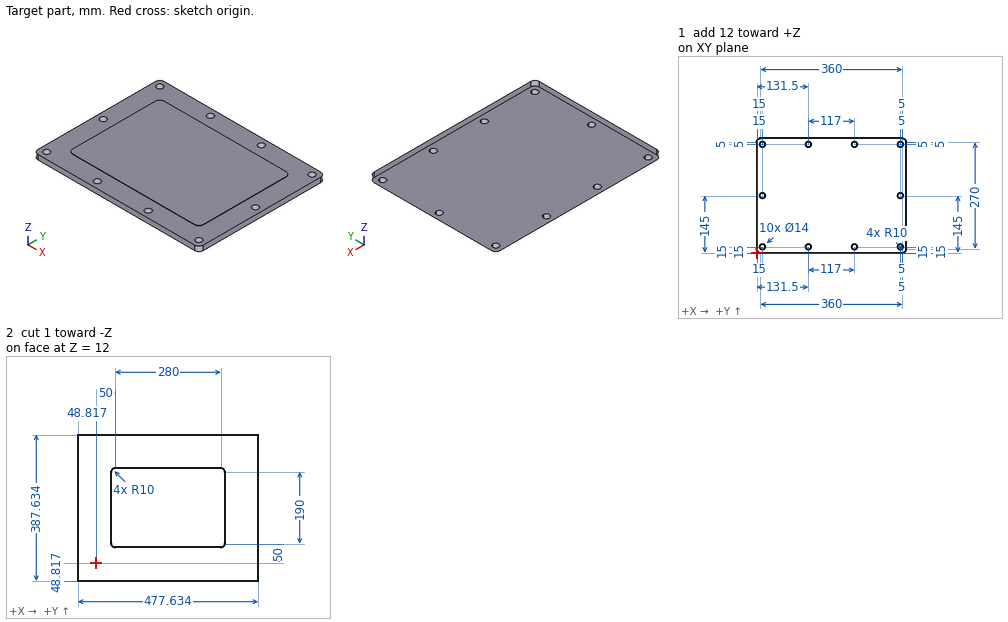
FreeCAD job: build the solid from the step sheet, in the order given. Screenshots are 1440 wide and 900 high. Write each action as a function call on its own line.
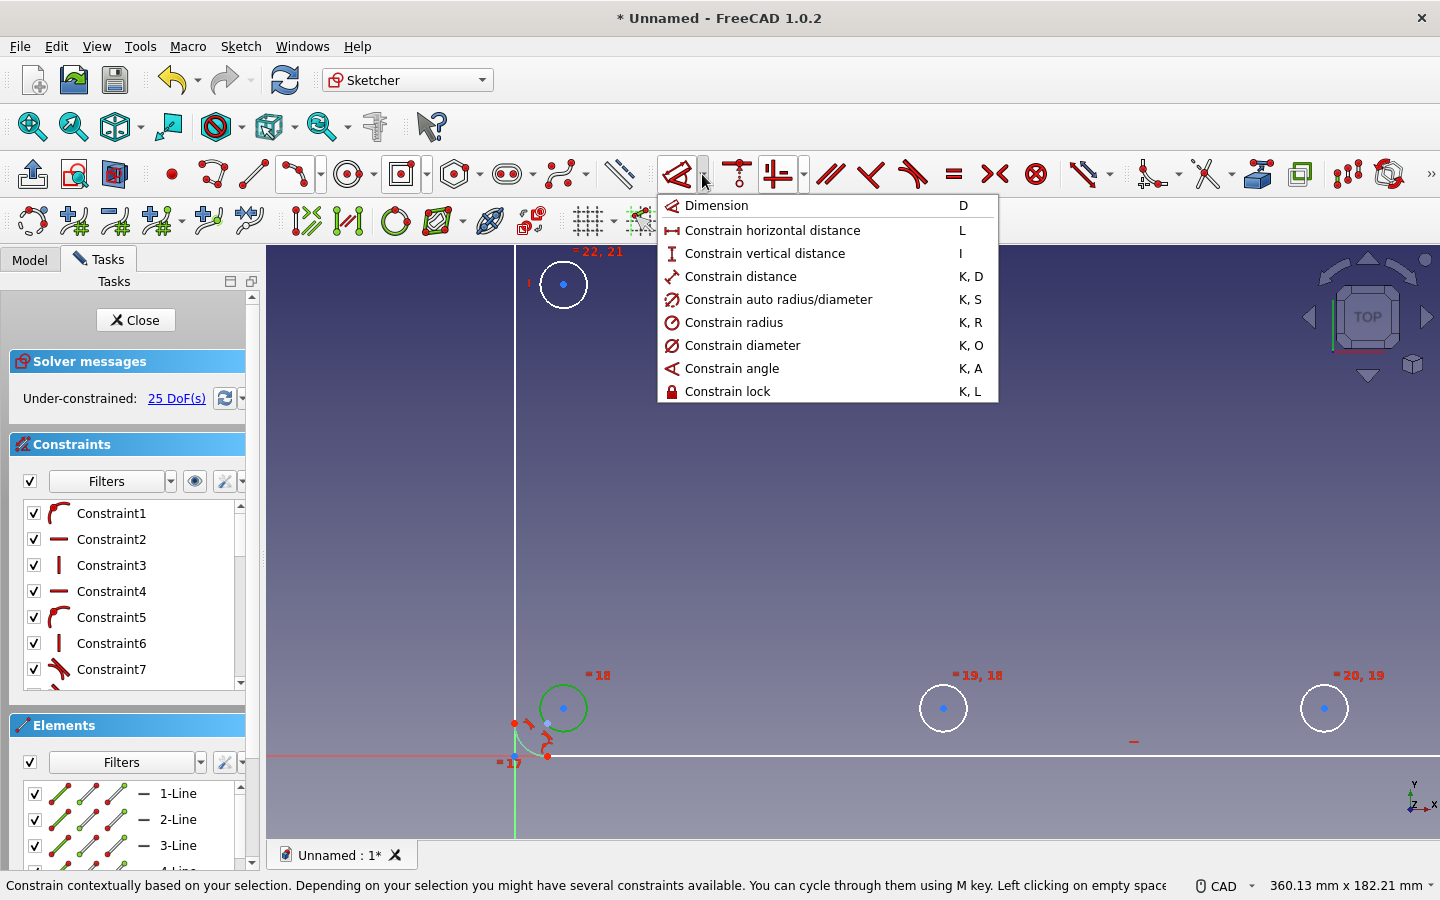
click(828, 346)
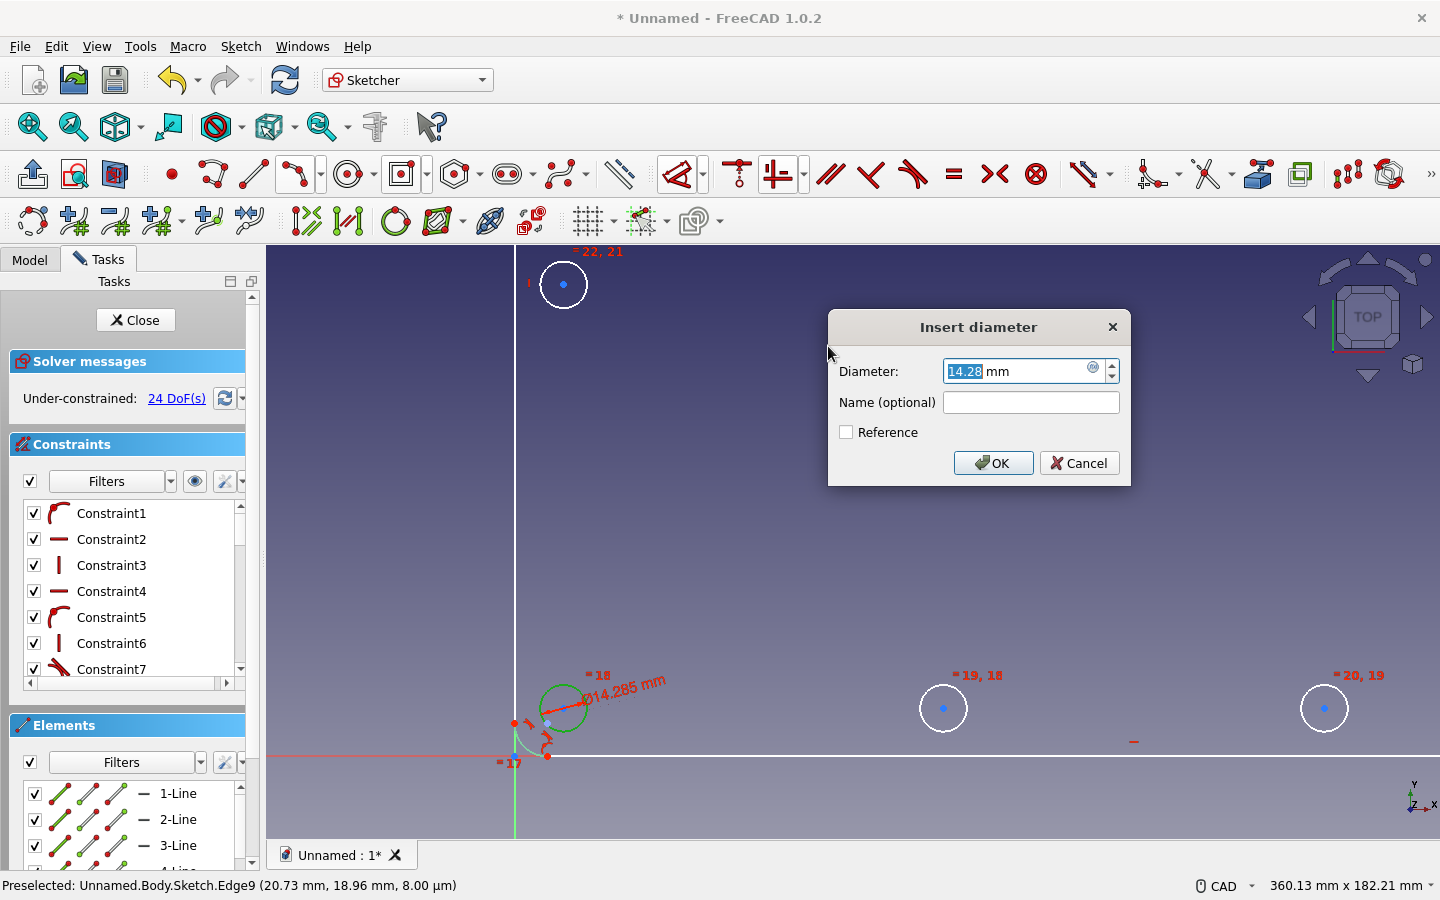
text(14)
key(Return)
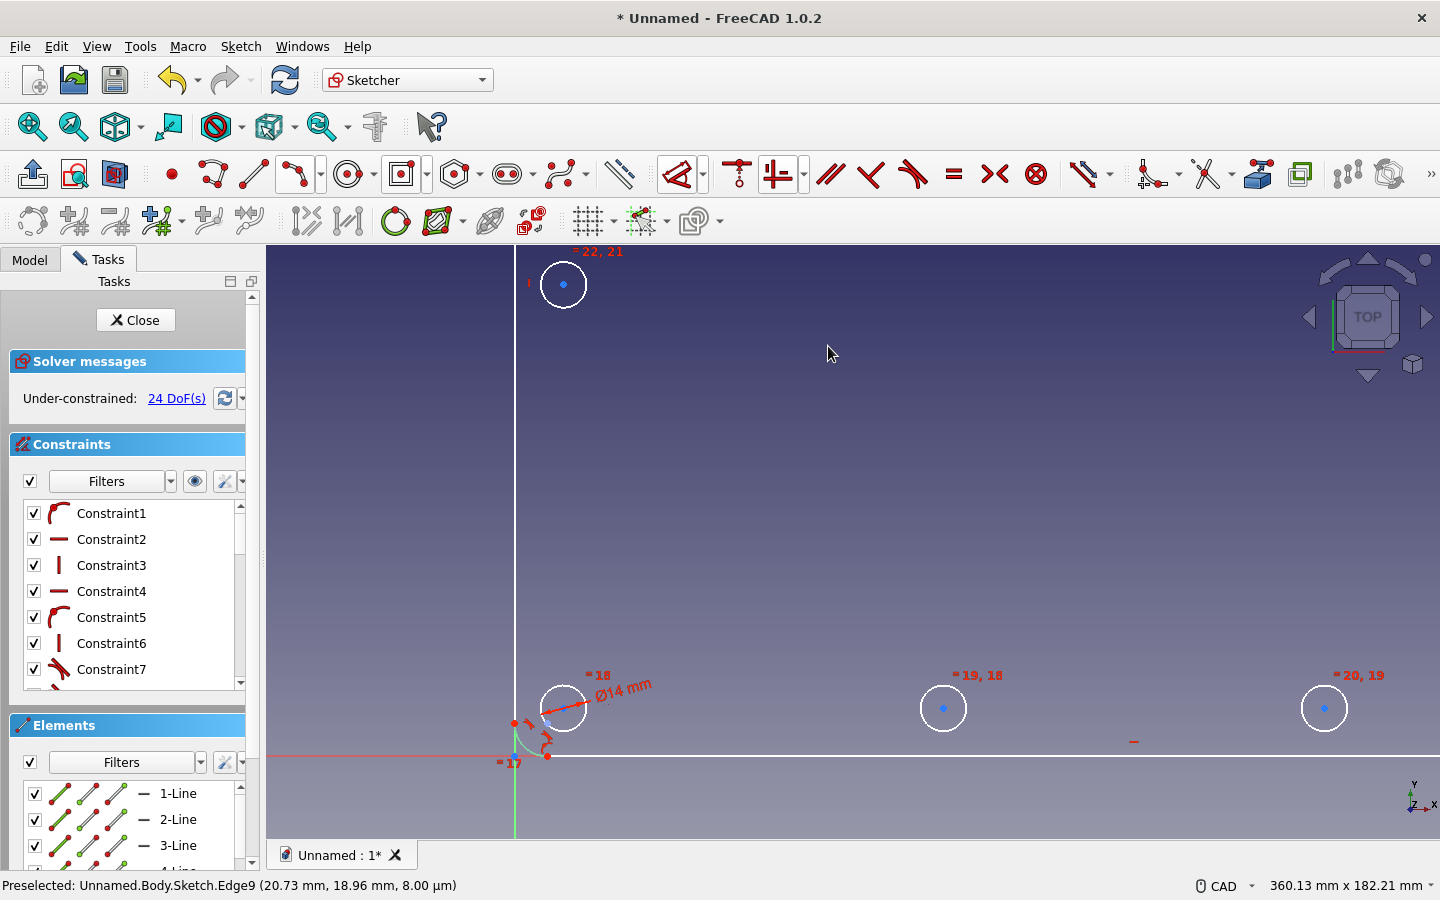
click(564, 708)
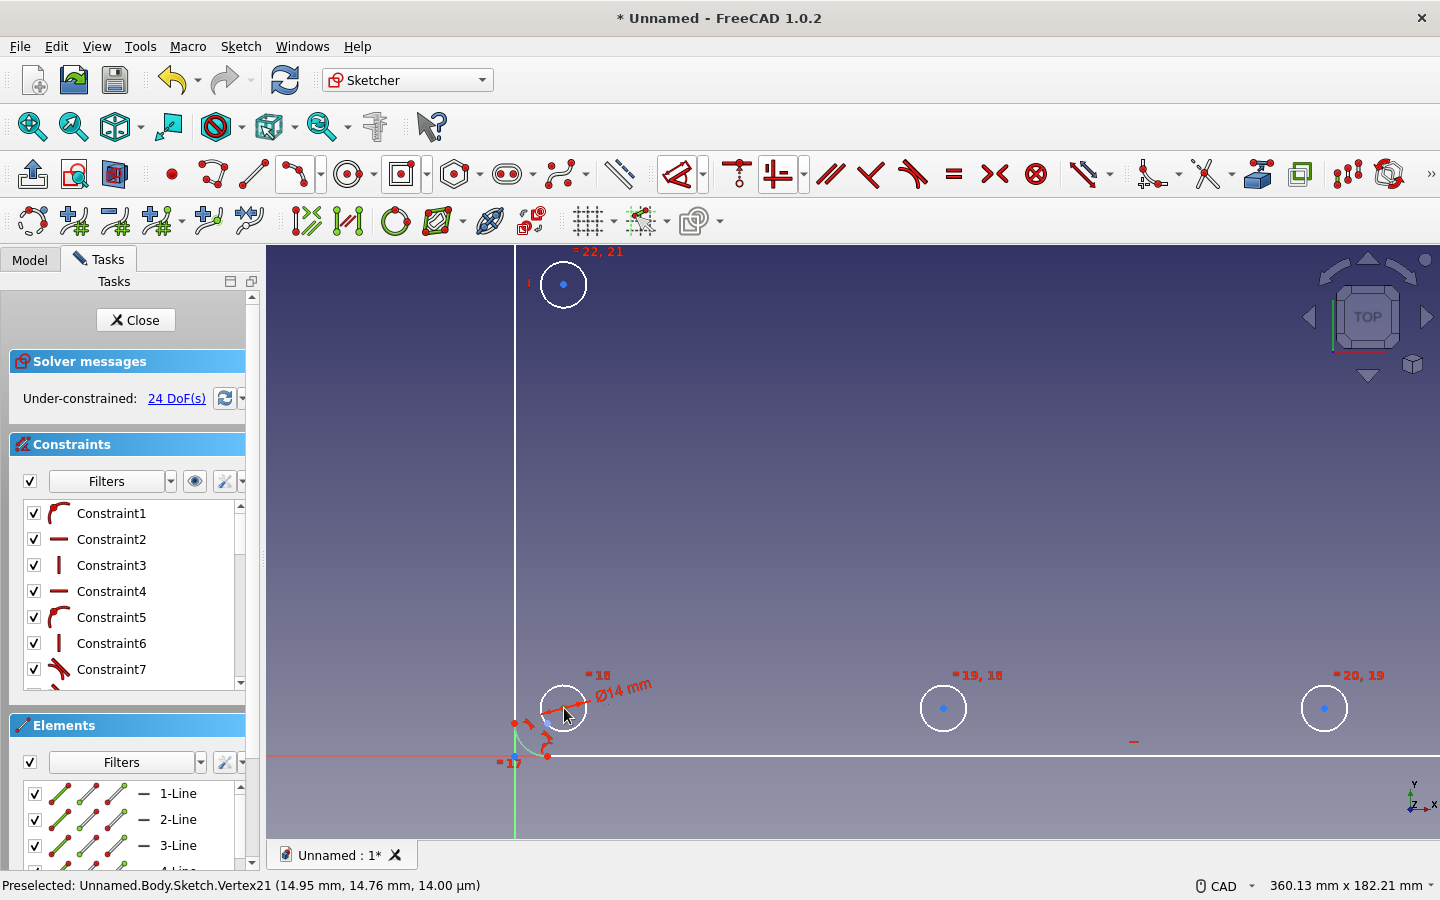
click(702, 174)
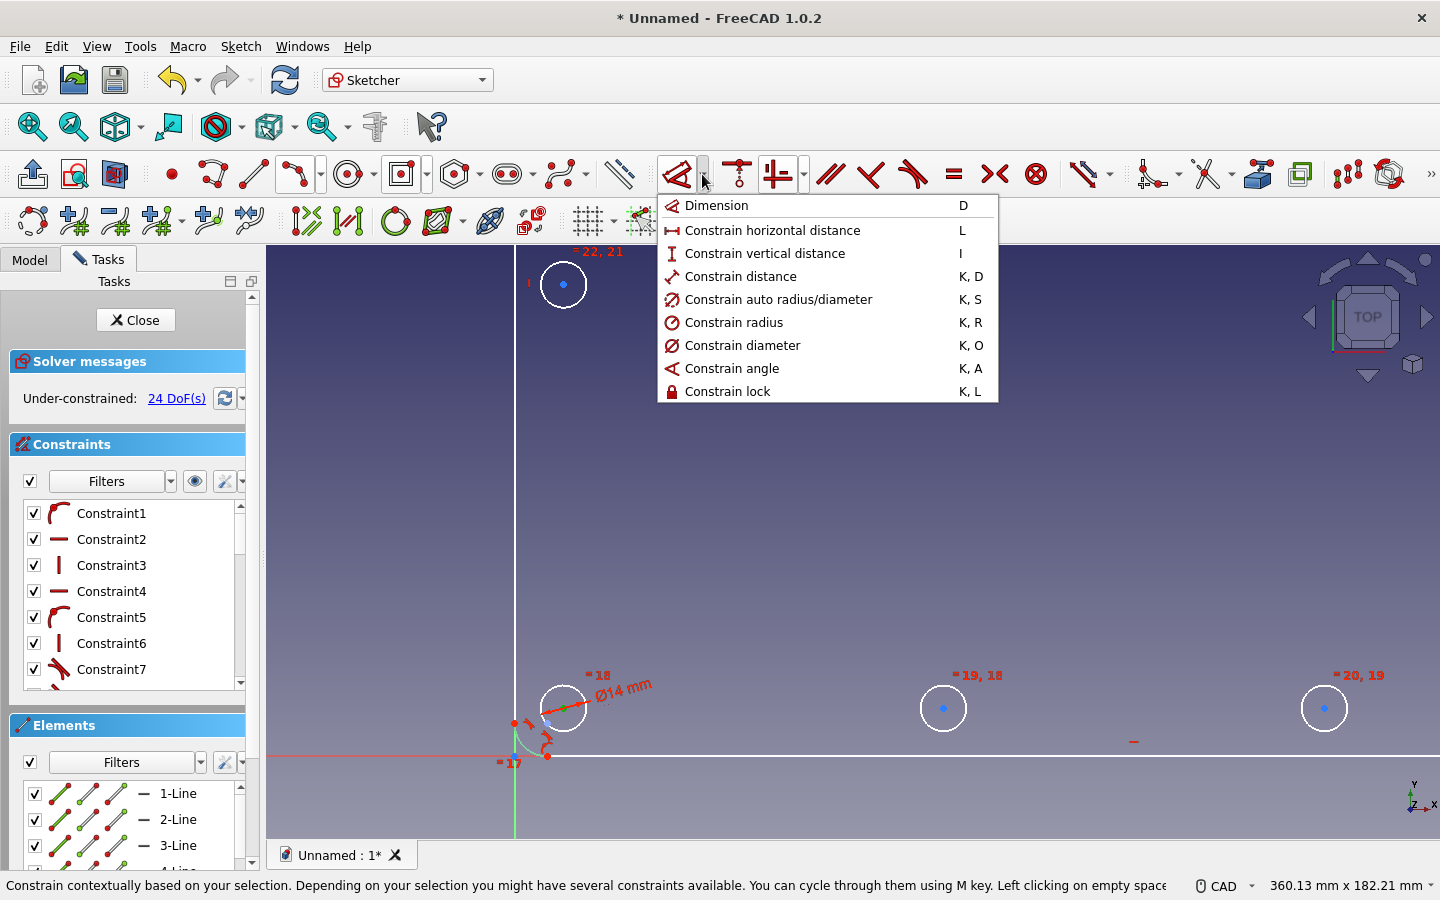
click(828, 230)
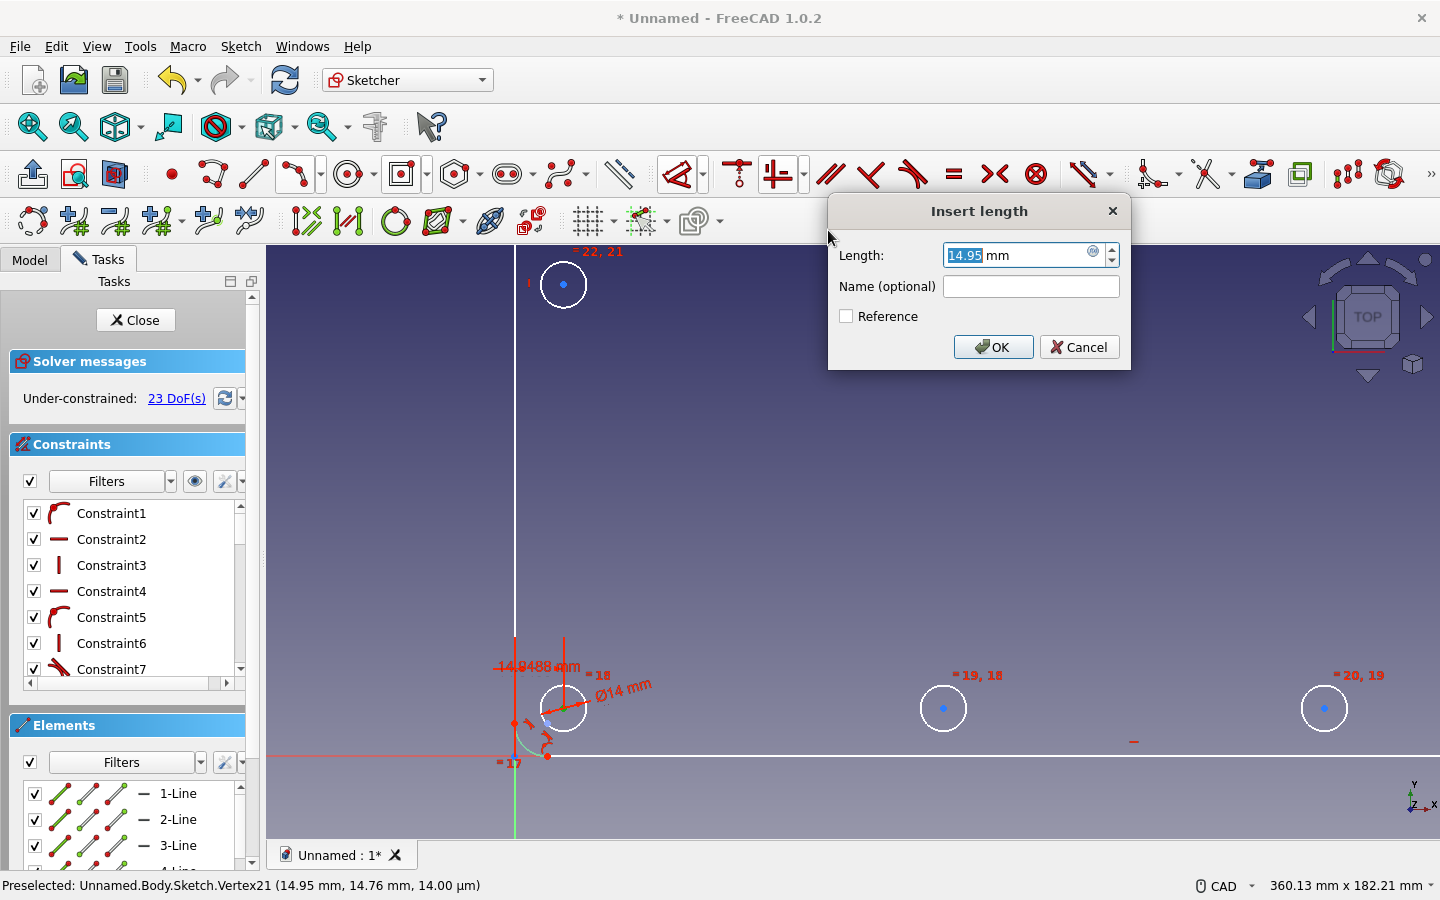
text(15)
key(Return)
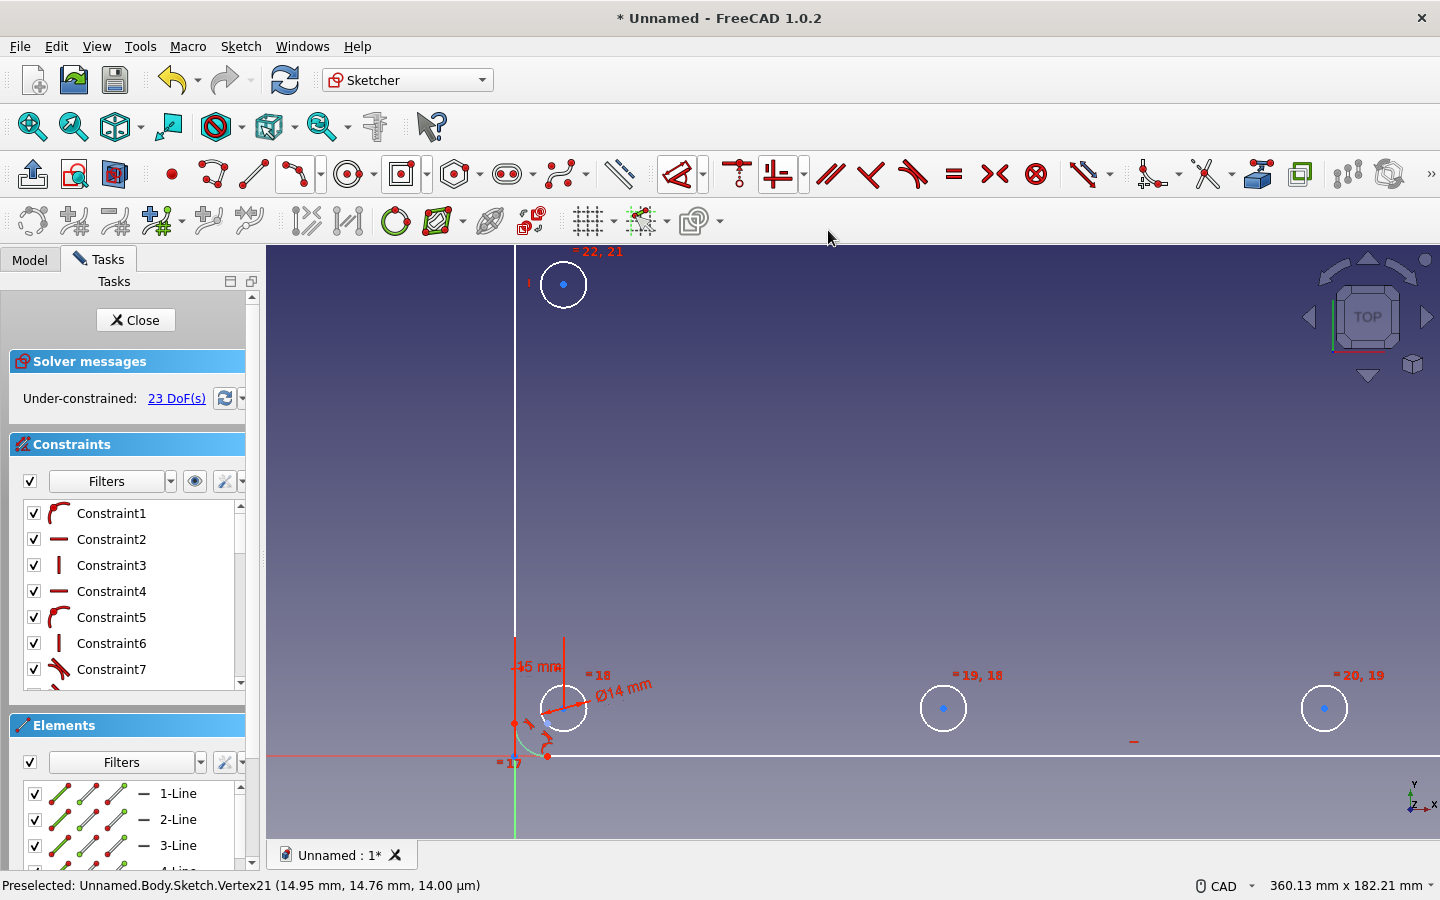
click(564, 708)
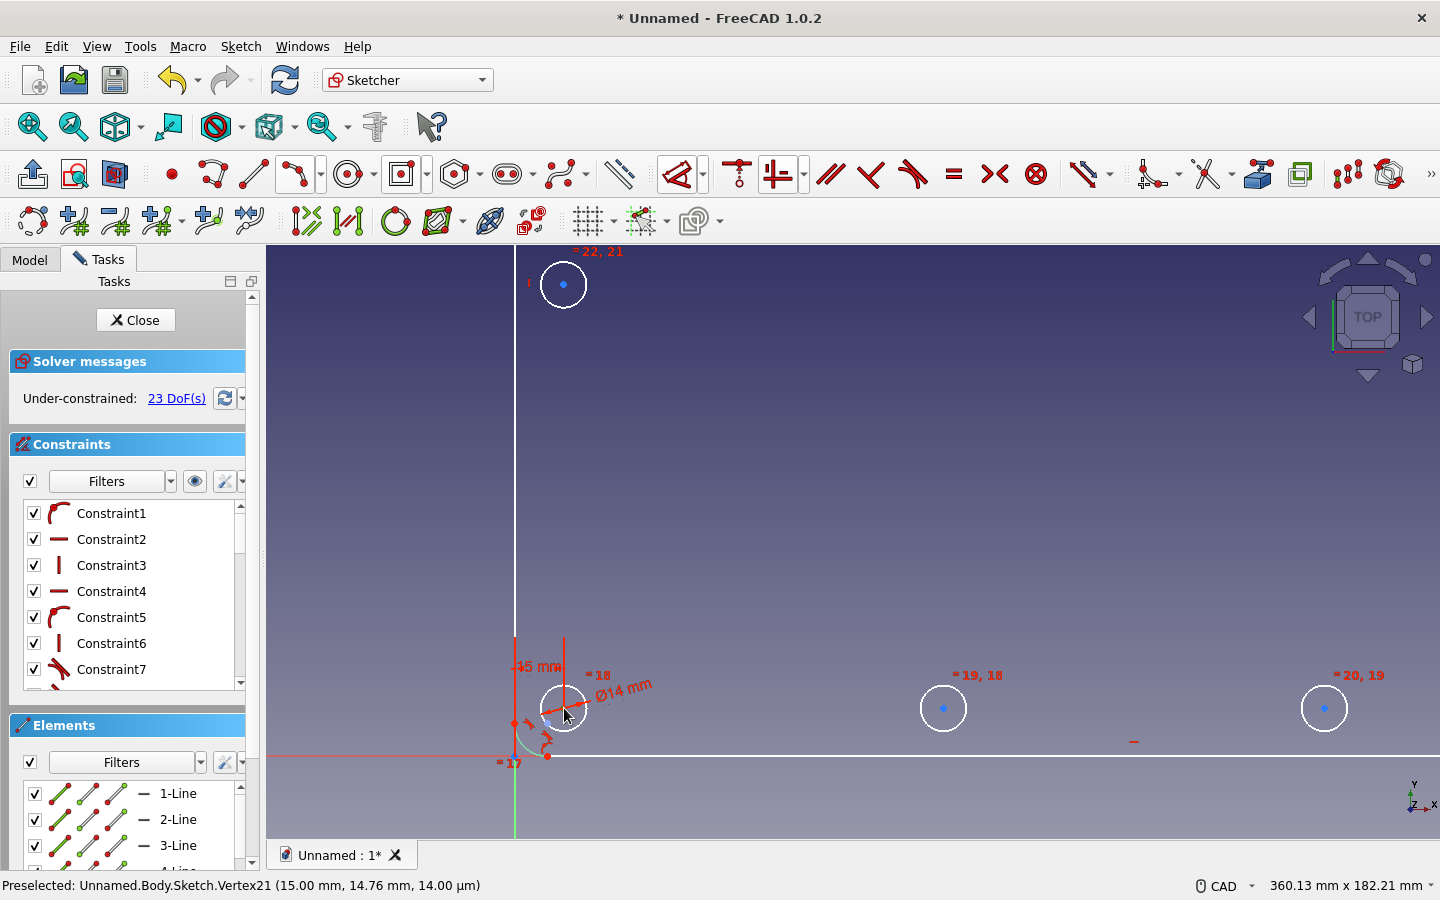
click(702, 174)